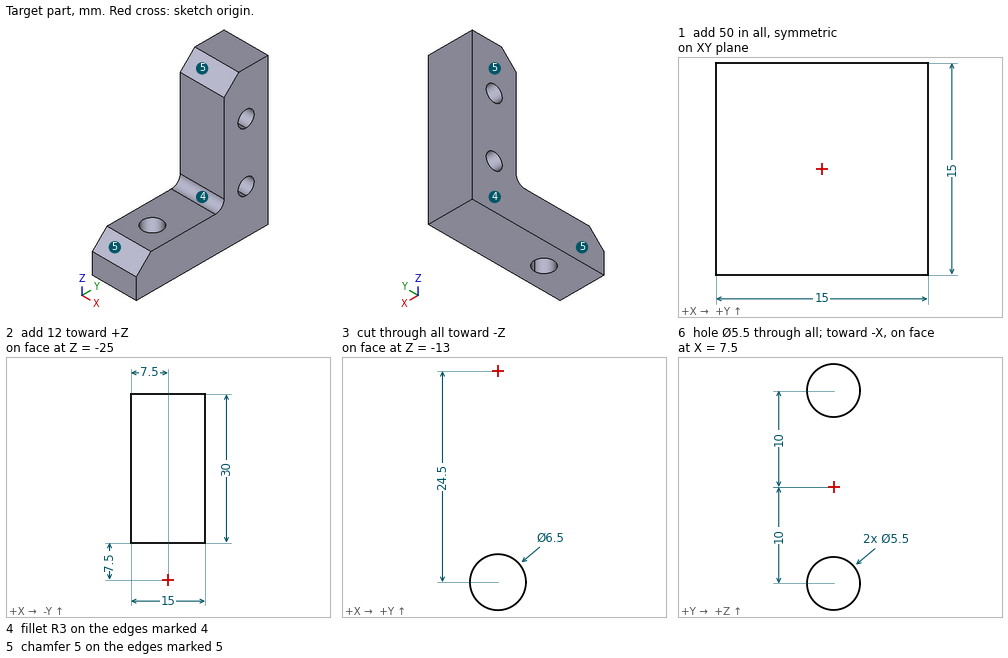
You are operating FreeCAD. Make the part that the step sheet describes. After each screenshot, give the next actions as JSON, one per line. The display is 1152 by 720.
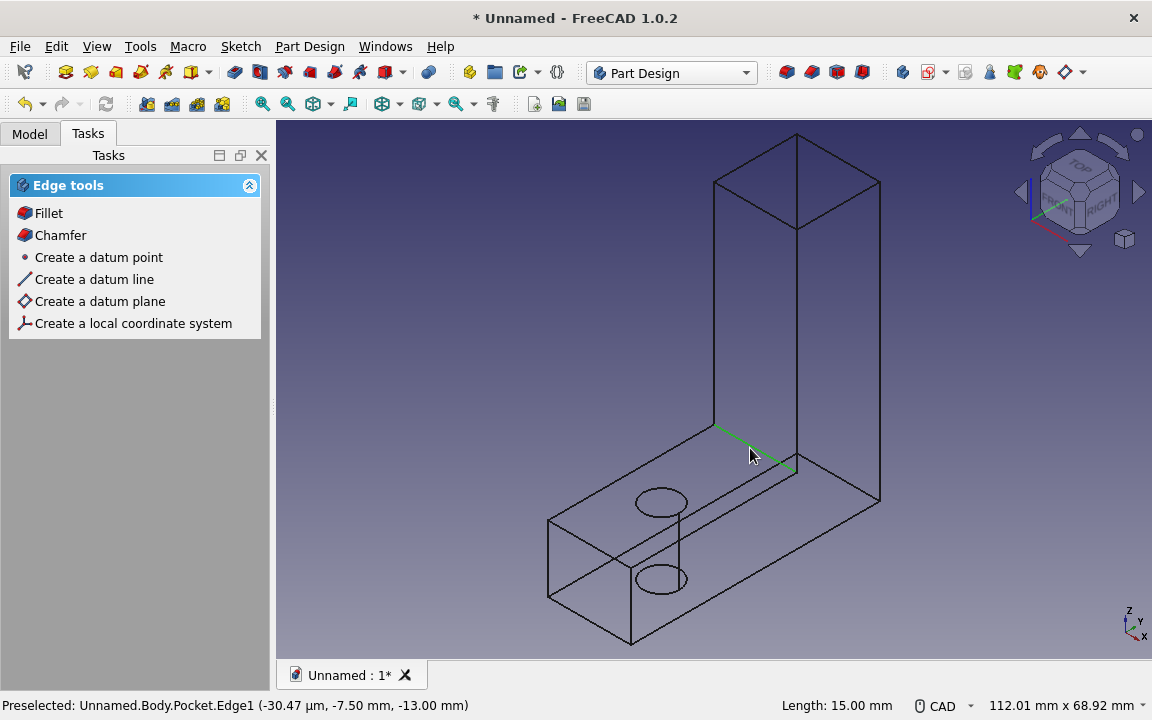
{"action": "key", "text": "v 1"}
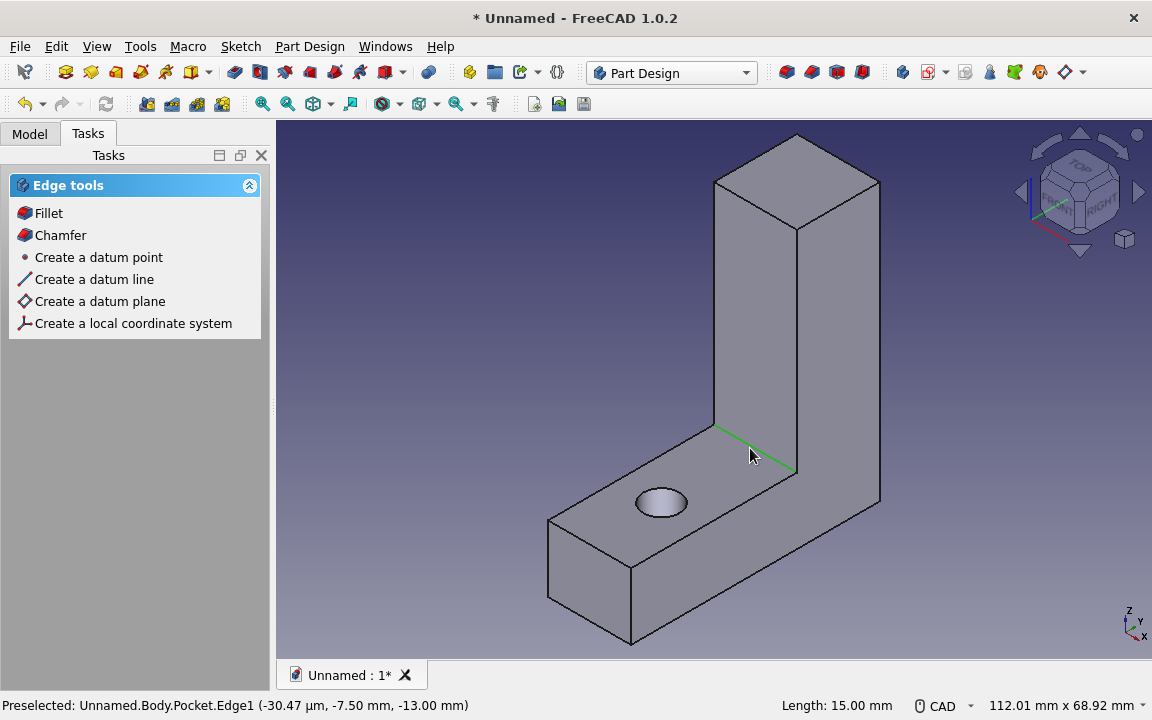
{"action": "left_click", "coordinate": [787, 72]}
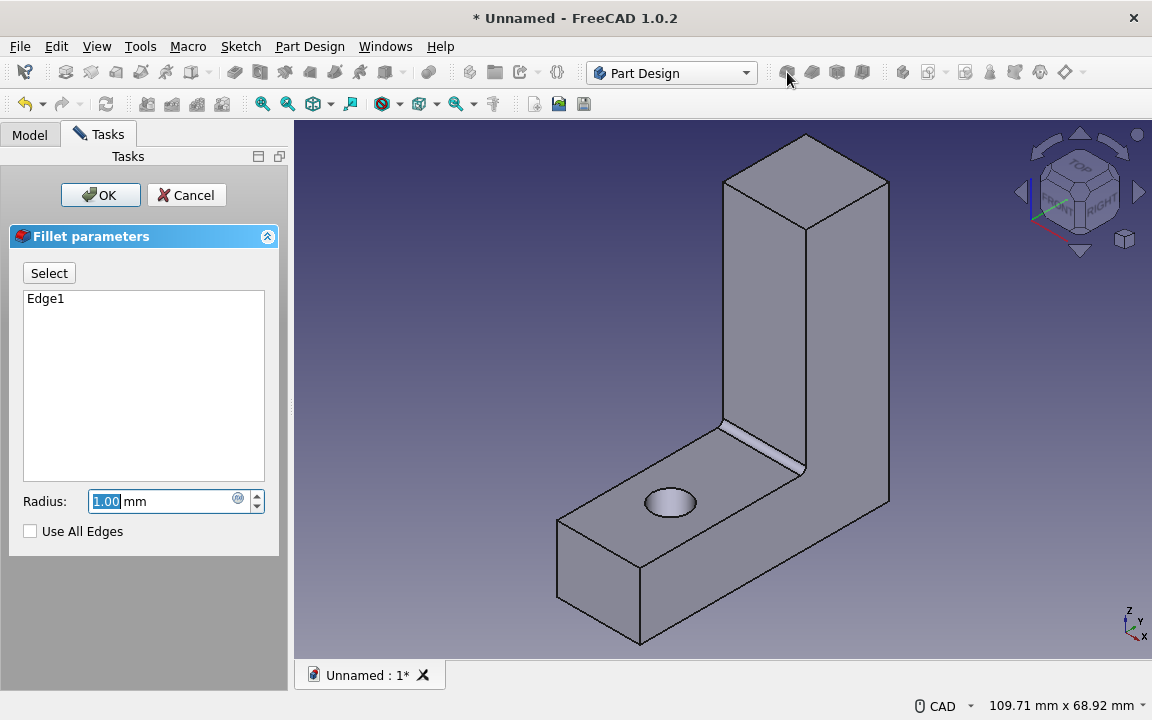
{"action": "type", "text": "3"}
{"action": "key", "text": "Tab"}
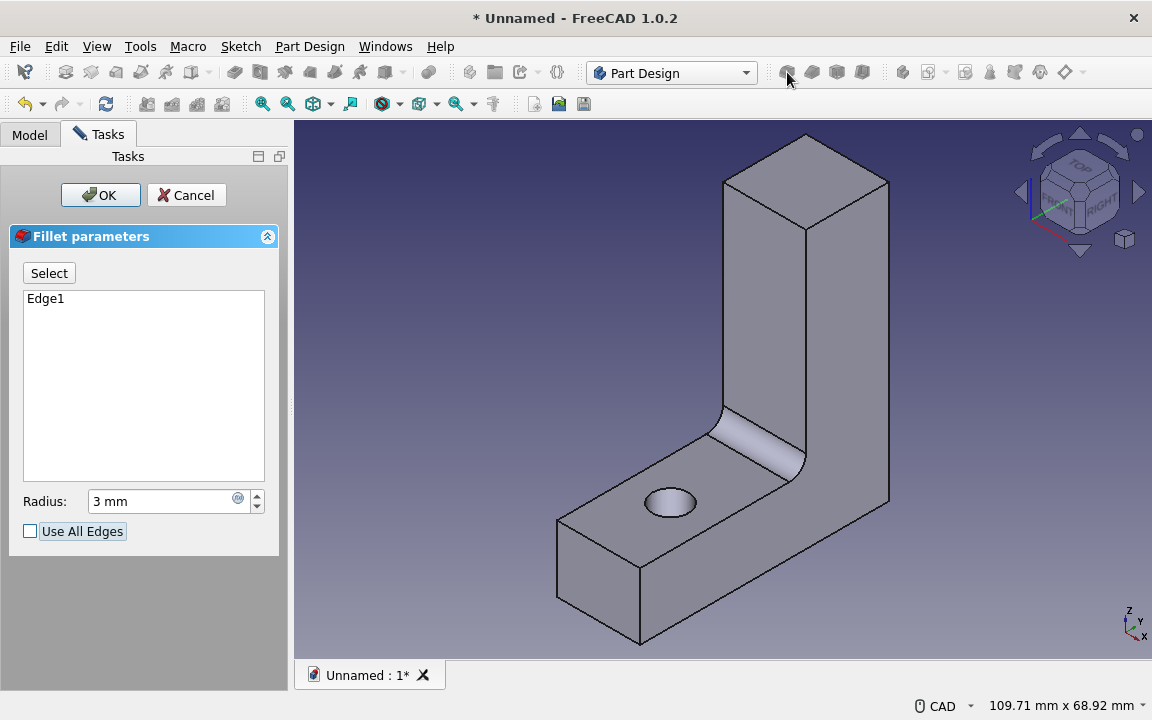
{"action": "left_click", "coordinate": [101, 195]}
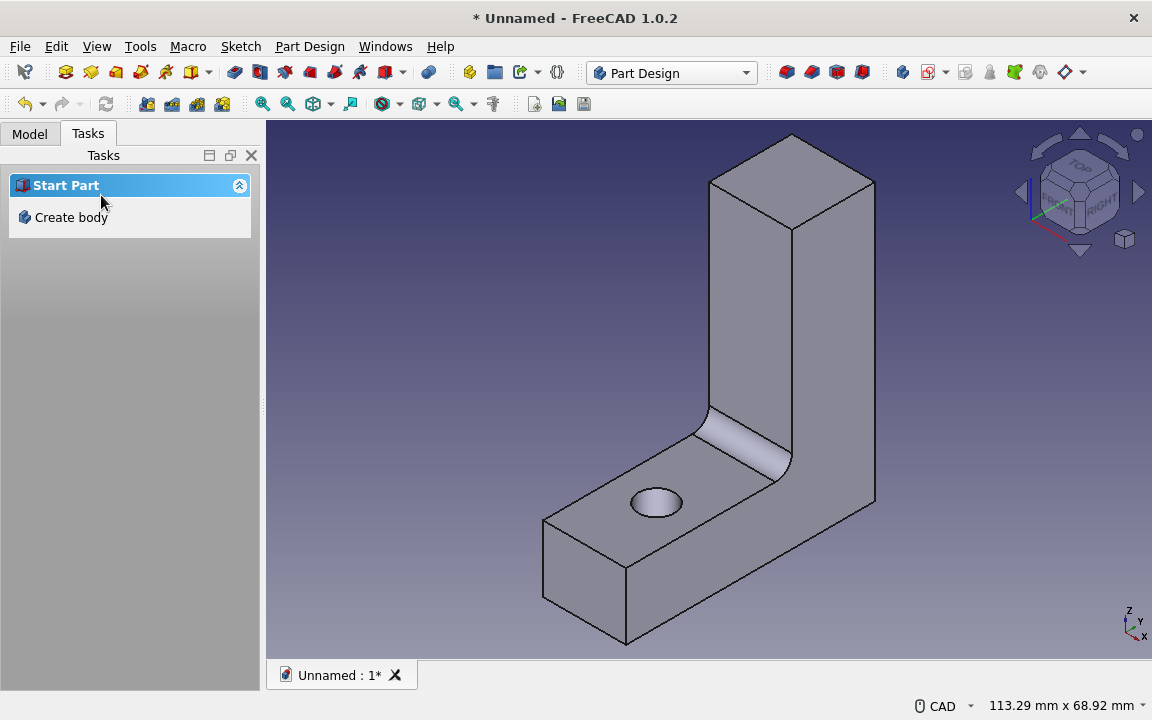
{"action": "left_click", "coordinate": [585, 543]}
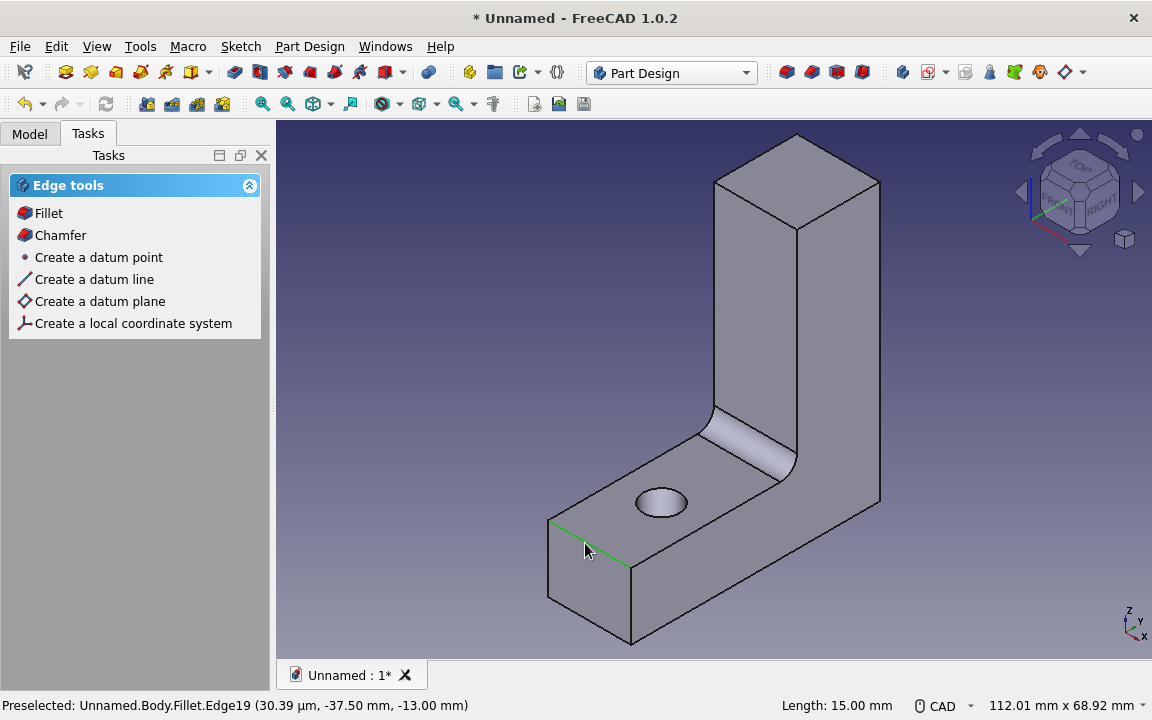
{"action": "left_click", "coordinate": [755, 205], "text": "ctrl"}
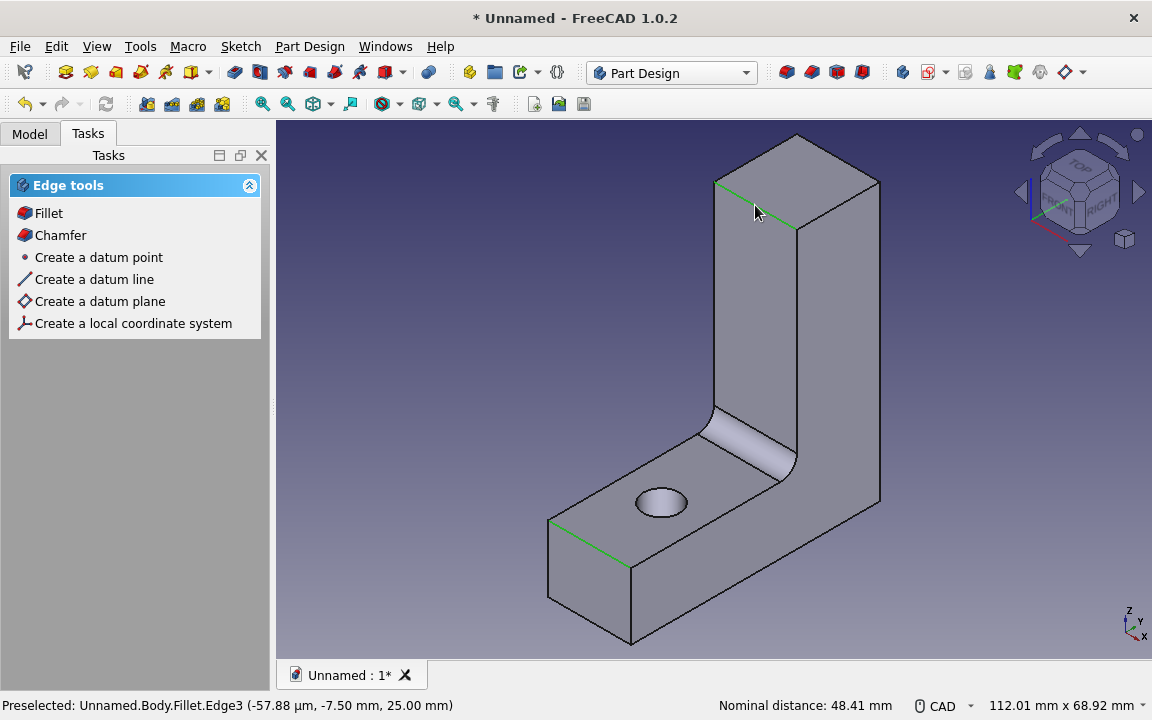
{"action": "left_click", "coordinate": [812, 72]}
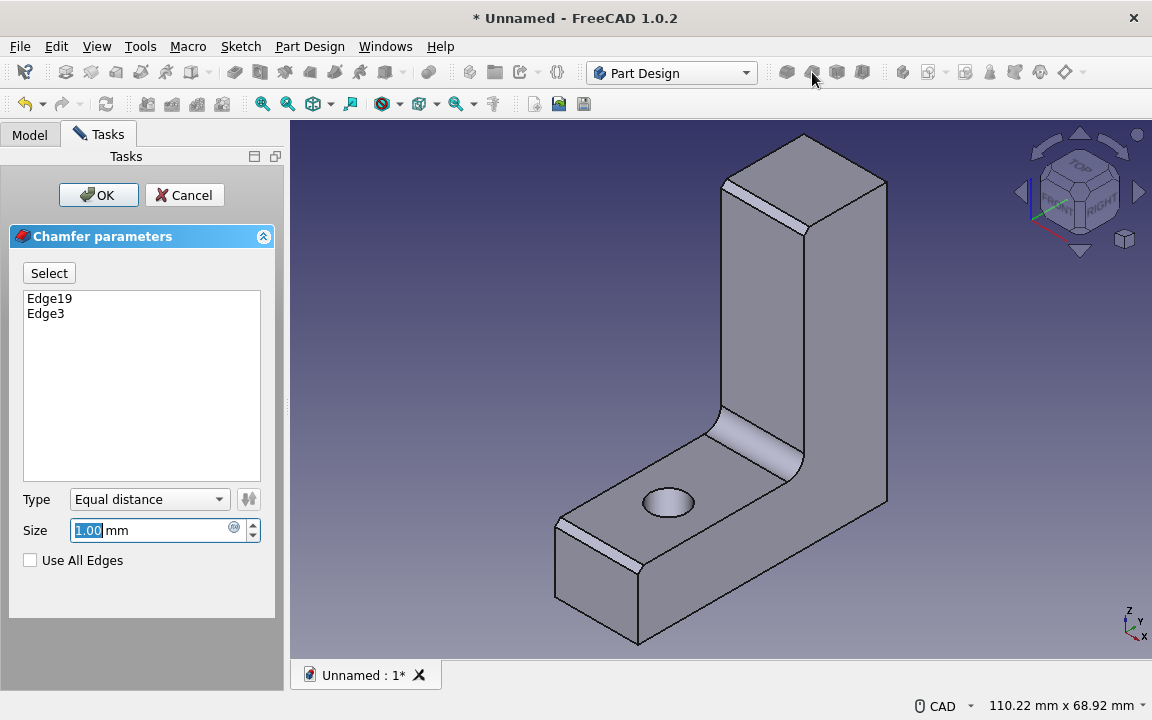
{"action": "type", "text": "5"}
{"action": "key", "text": "Tab"}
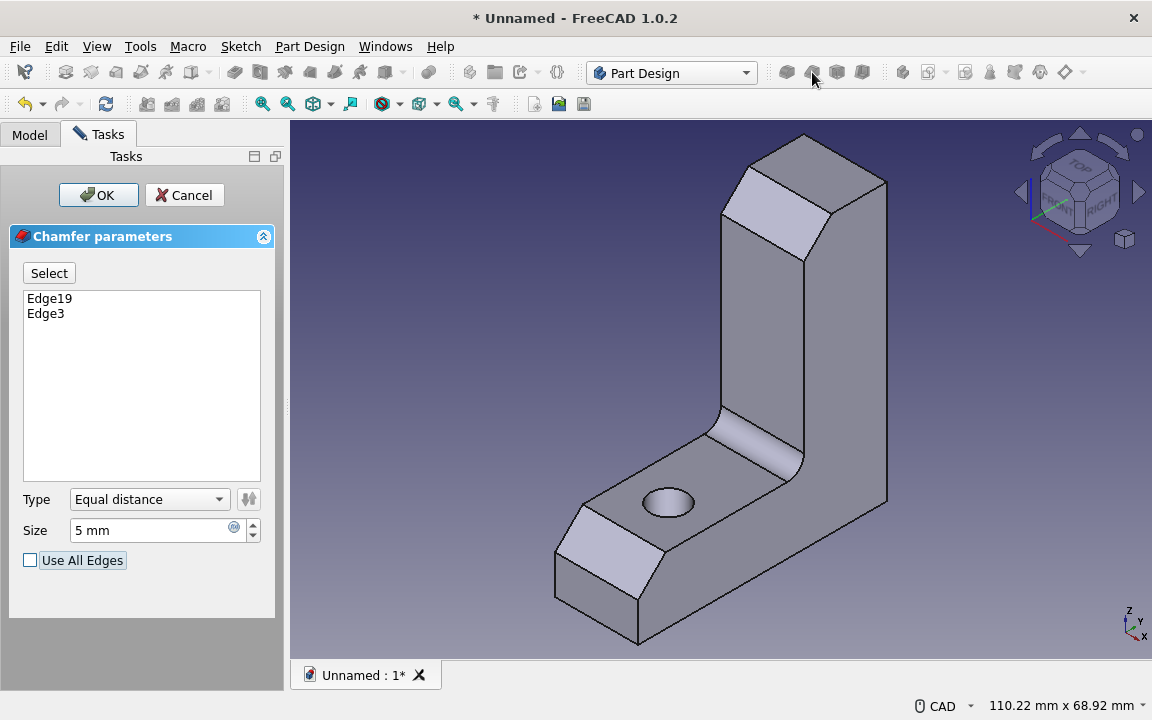
{"action": "left_click", "coordinate": [99, 195]}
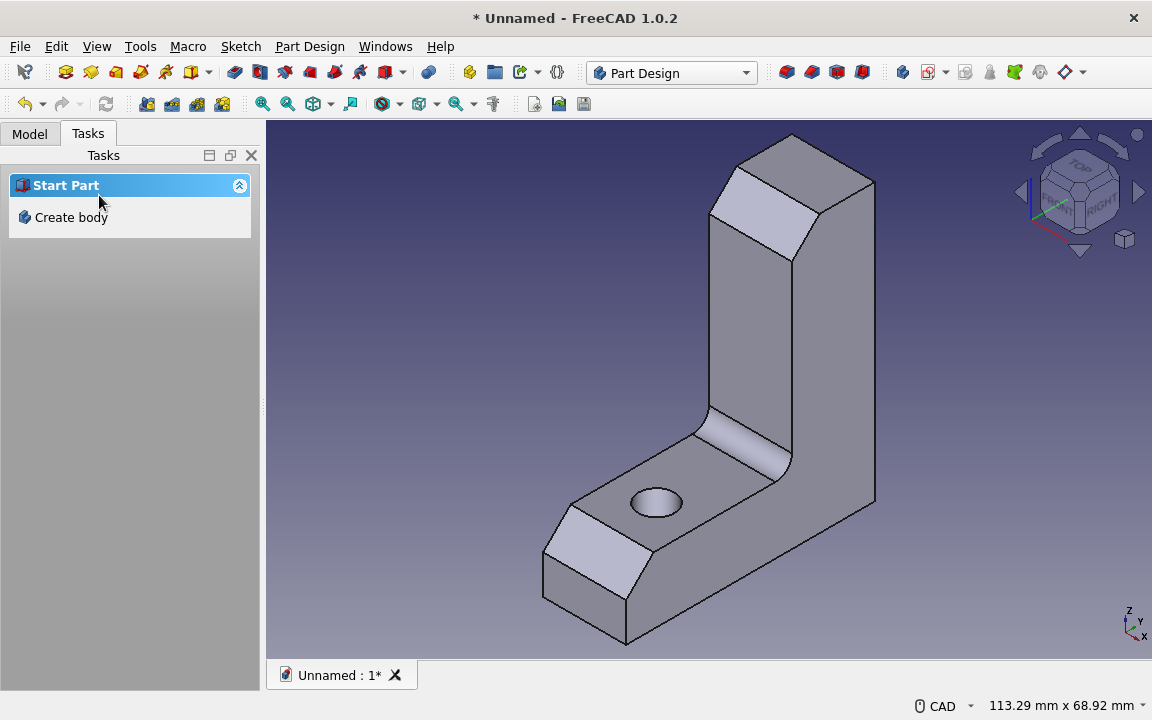
{"action": "left_click", "coordinate": [822, 463]}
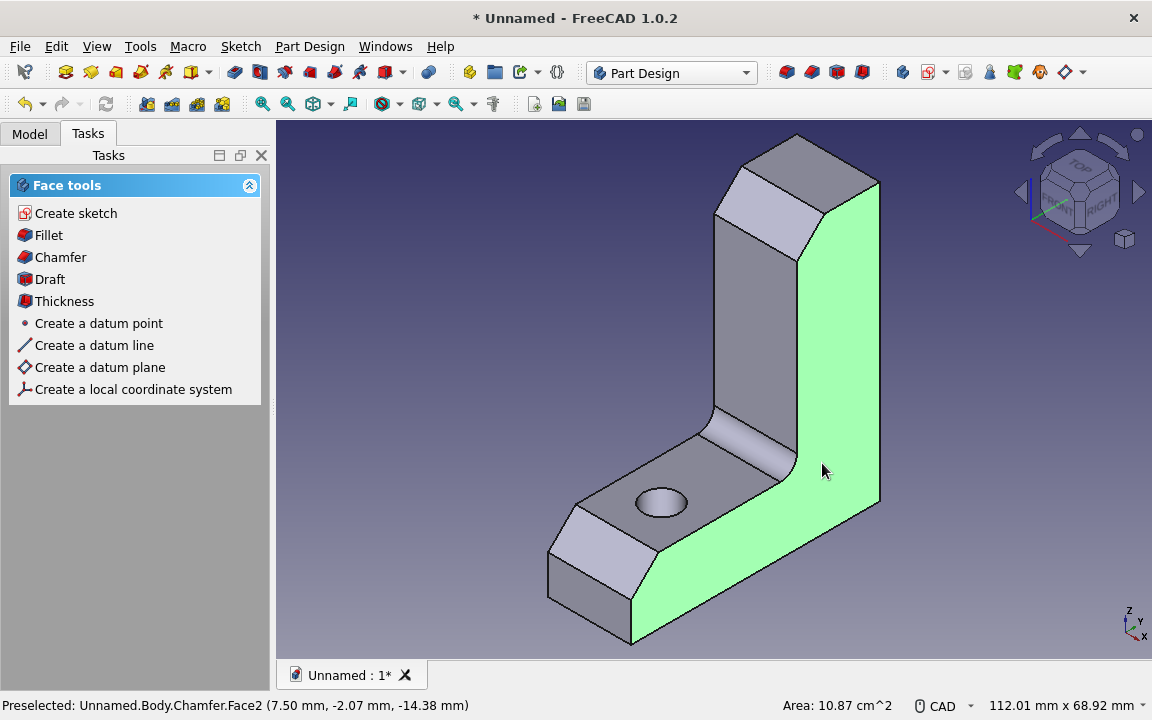
{"action": "left_click", "coordinate": [928, 72]}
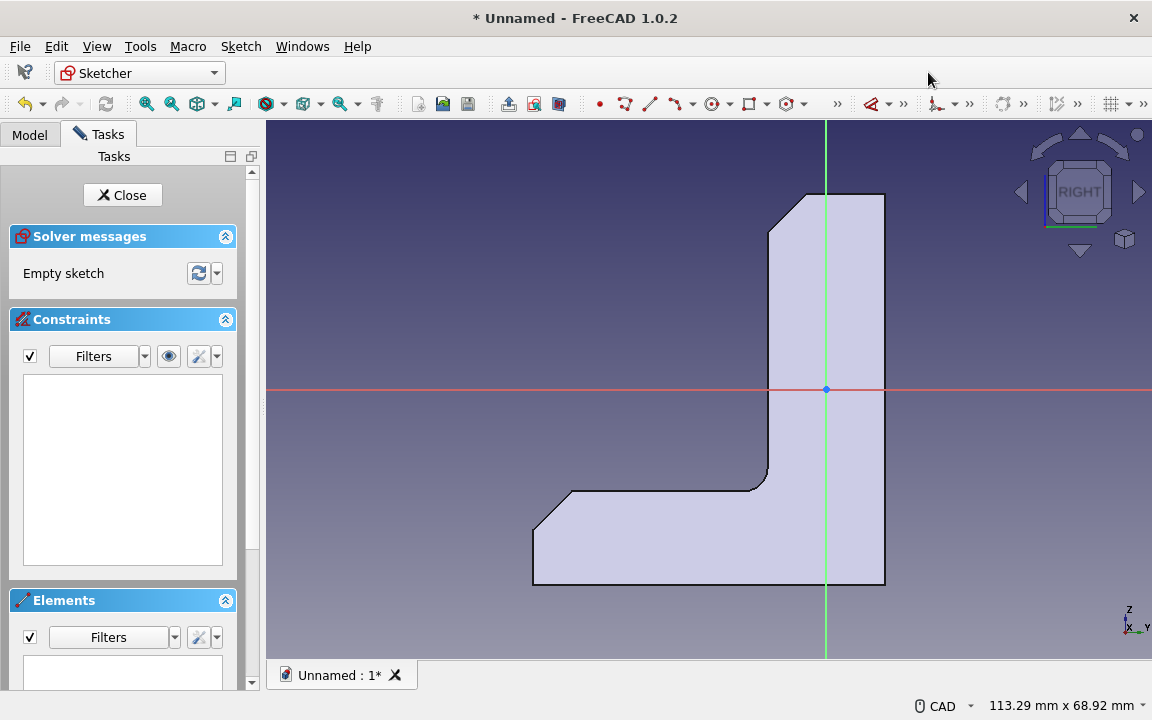
{"action": "scroll", "coordinate": [987, 389], "scroll_direction": "up", "scroll_amount": 3}